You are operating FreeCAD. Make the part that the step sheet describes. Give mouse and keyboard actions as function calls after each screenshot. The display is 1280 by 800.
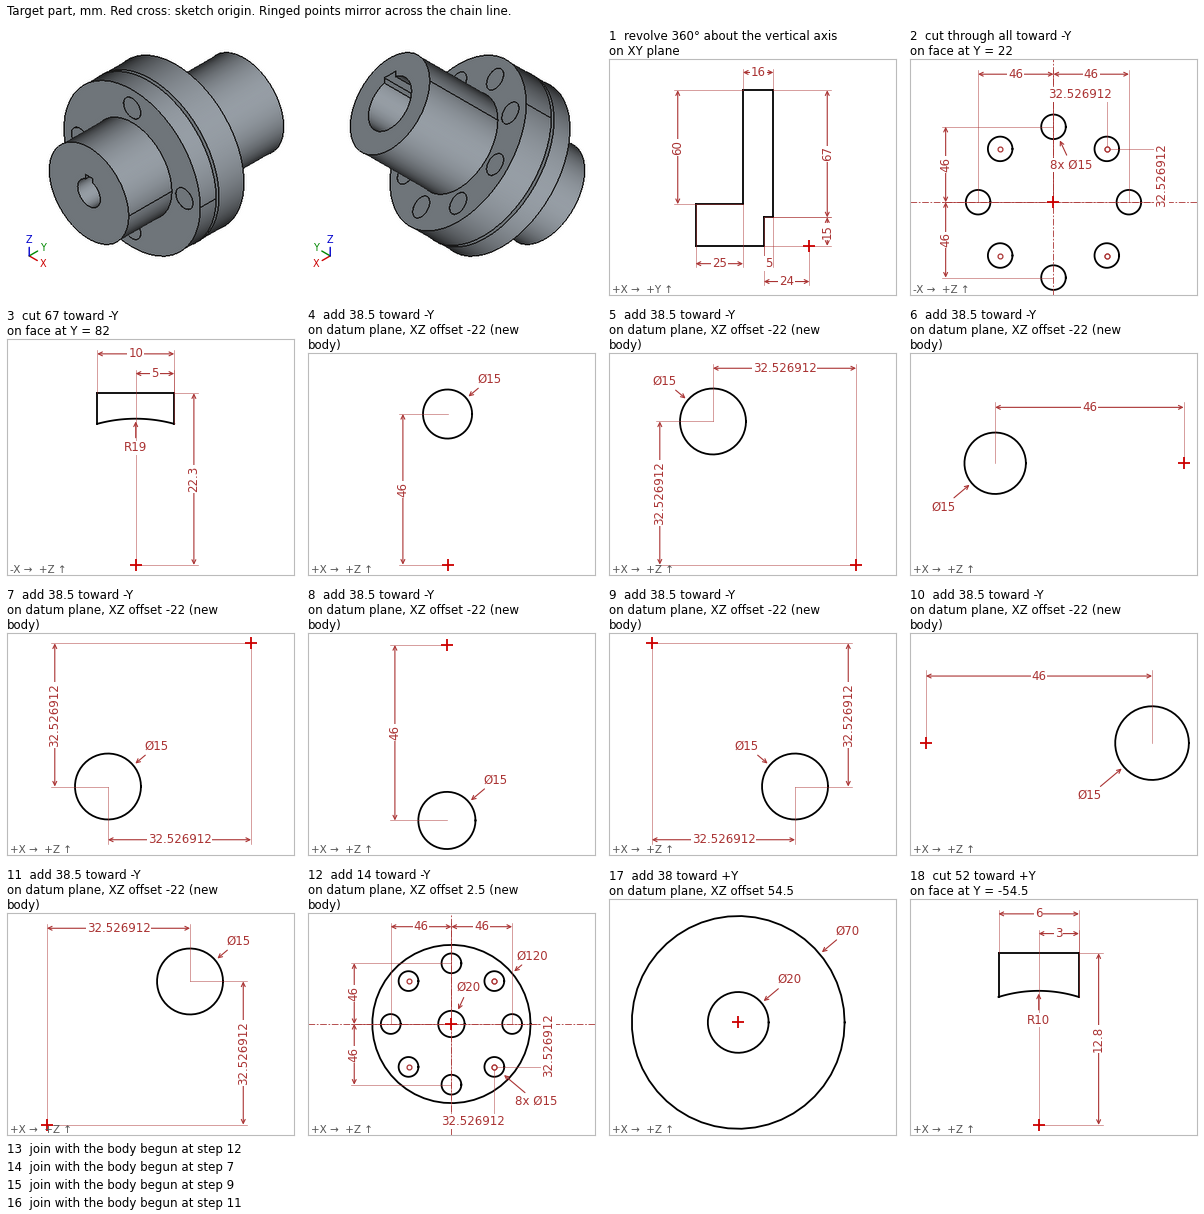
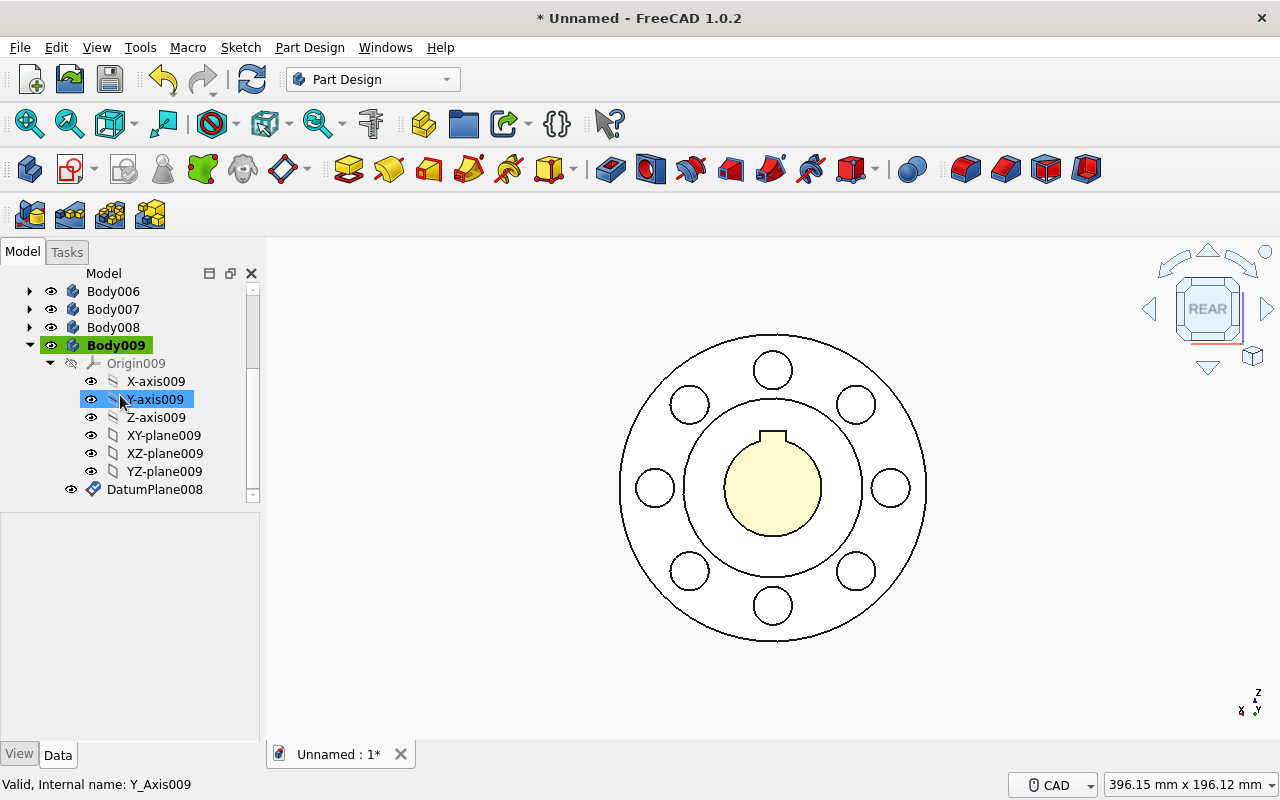
click(116, 489)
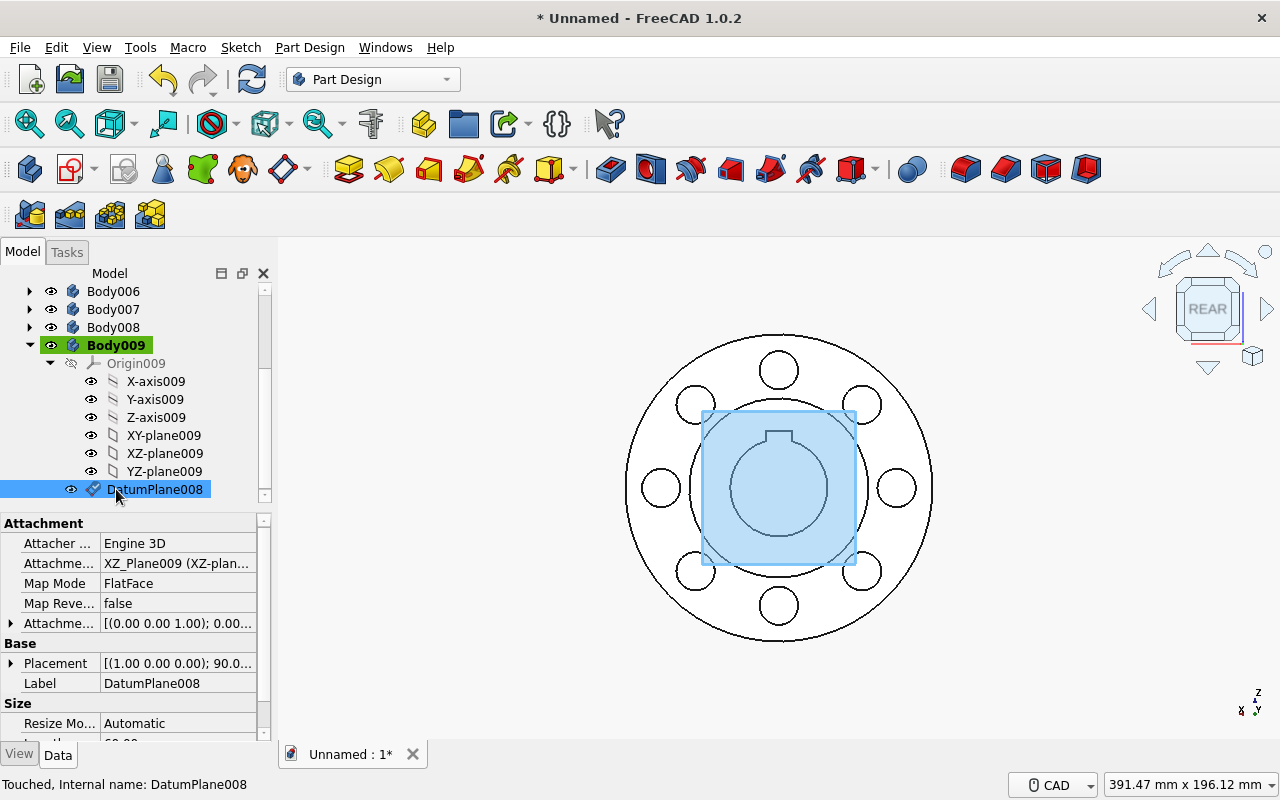
click(70, 170)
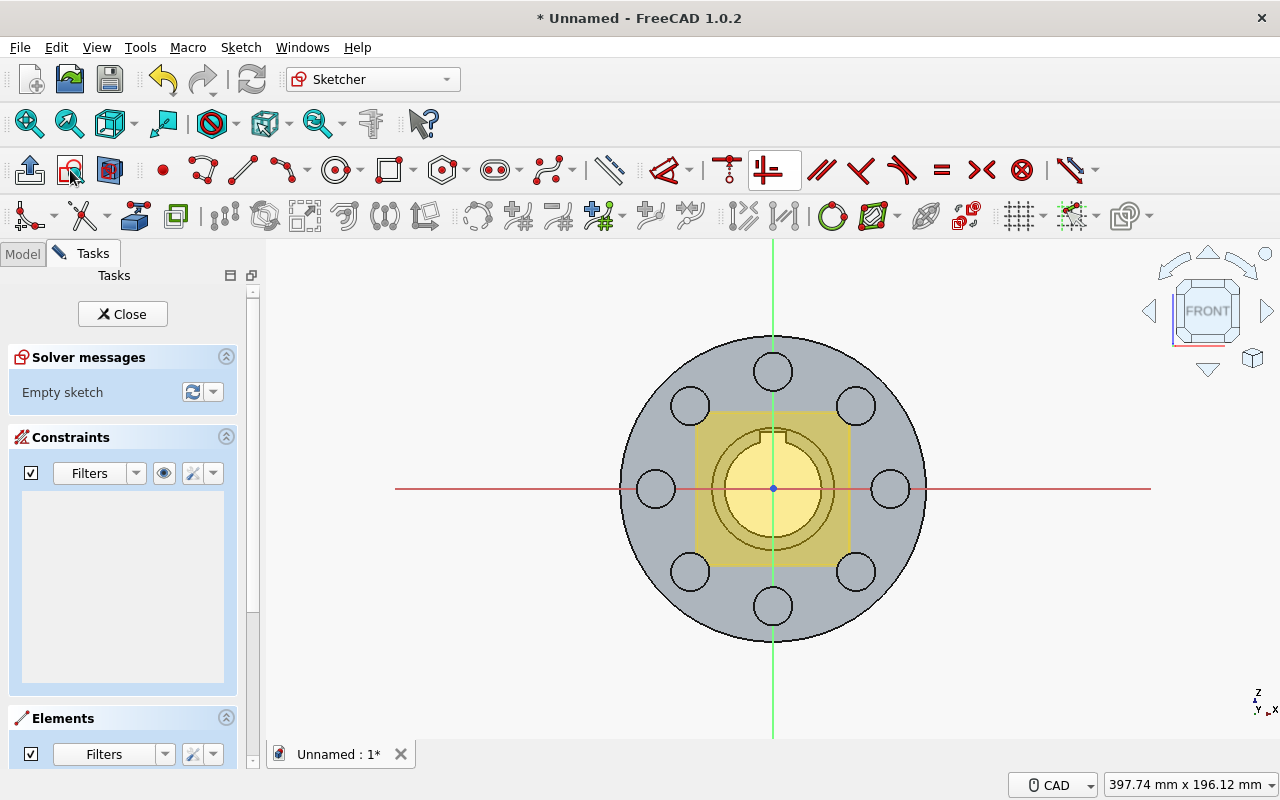
click(336, 170)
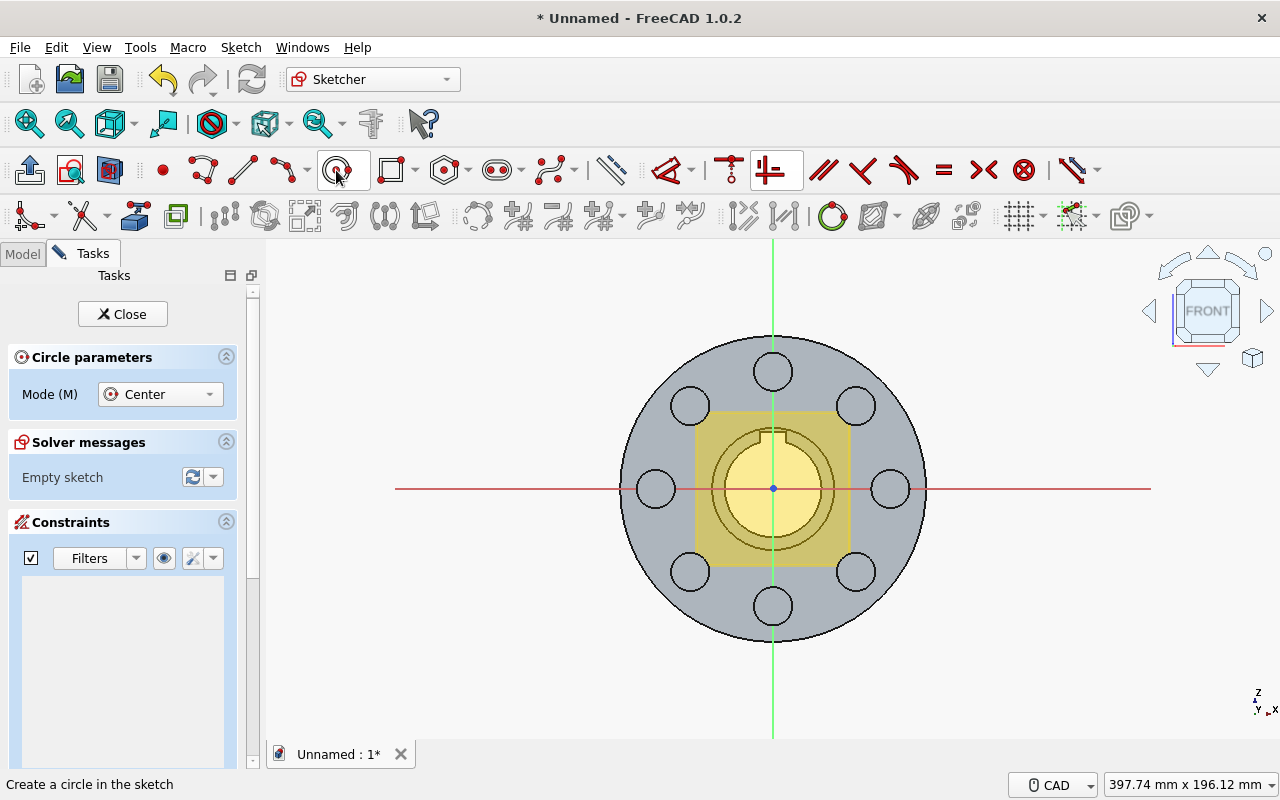
click(773, 489)
click(881, 381)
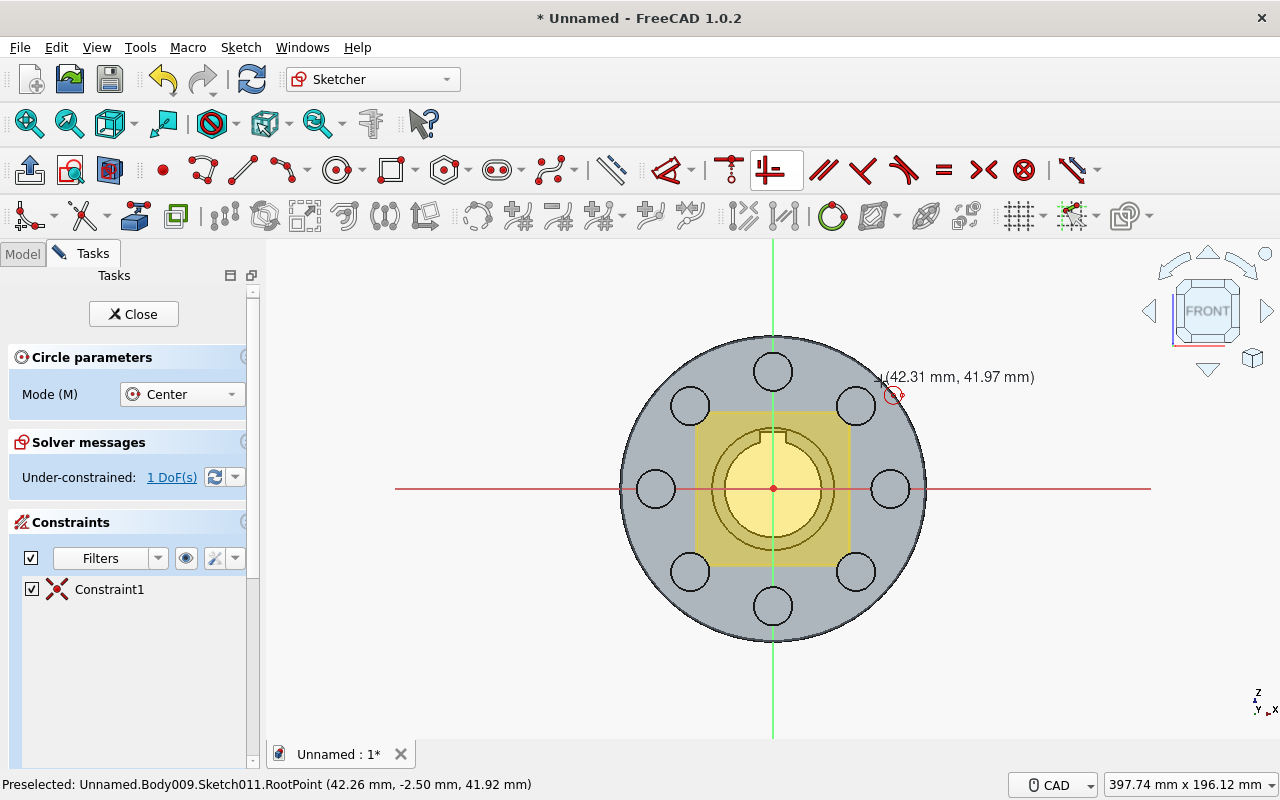
click(856, 572)
click(870, 558)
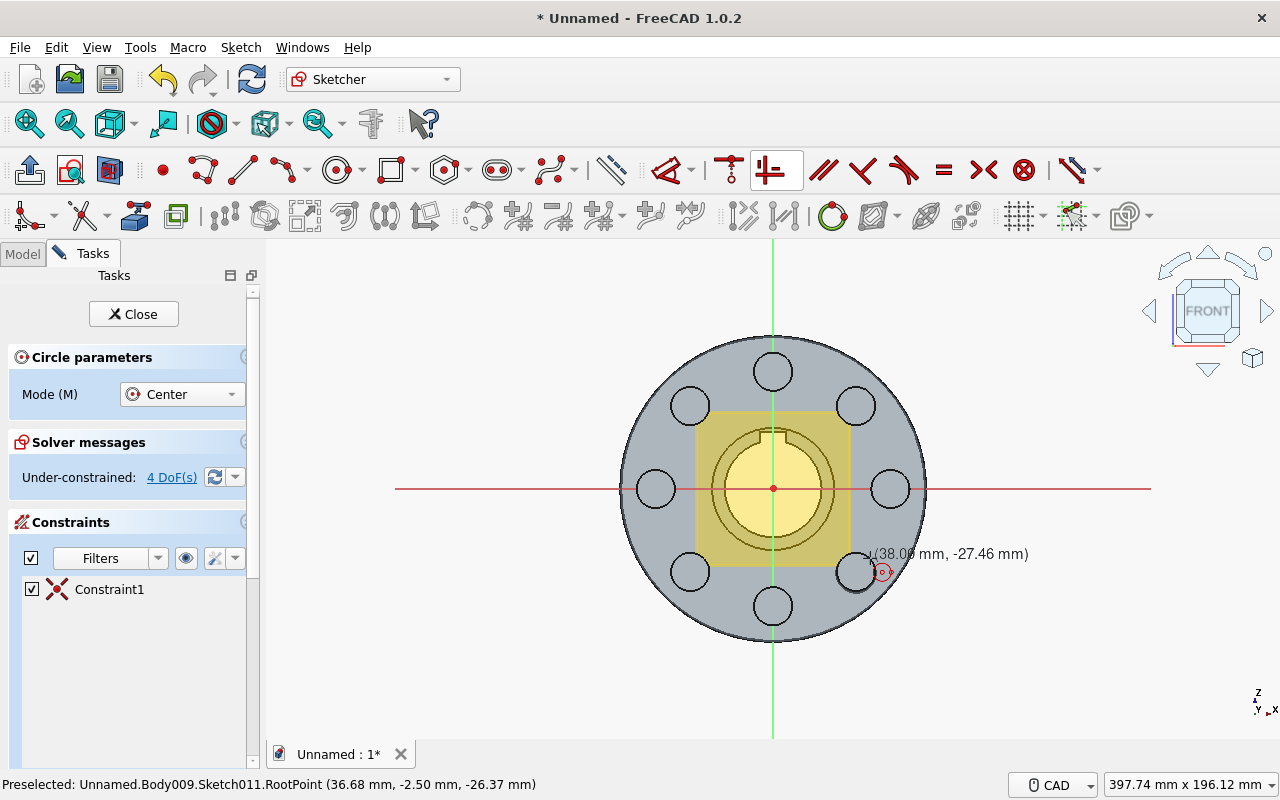
click(773, 606)
click(791, 600)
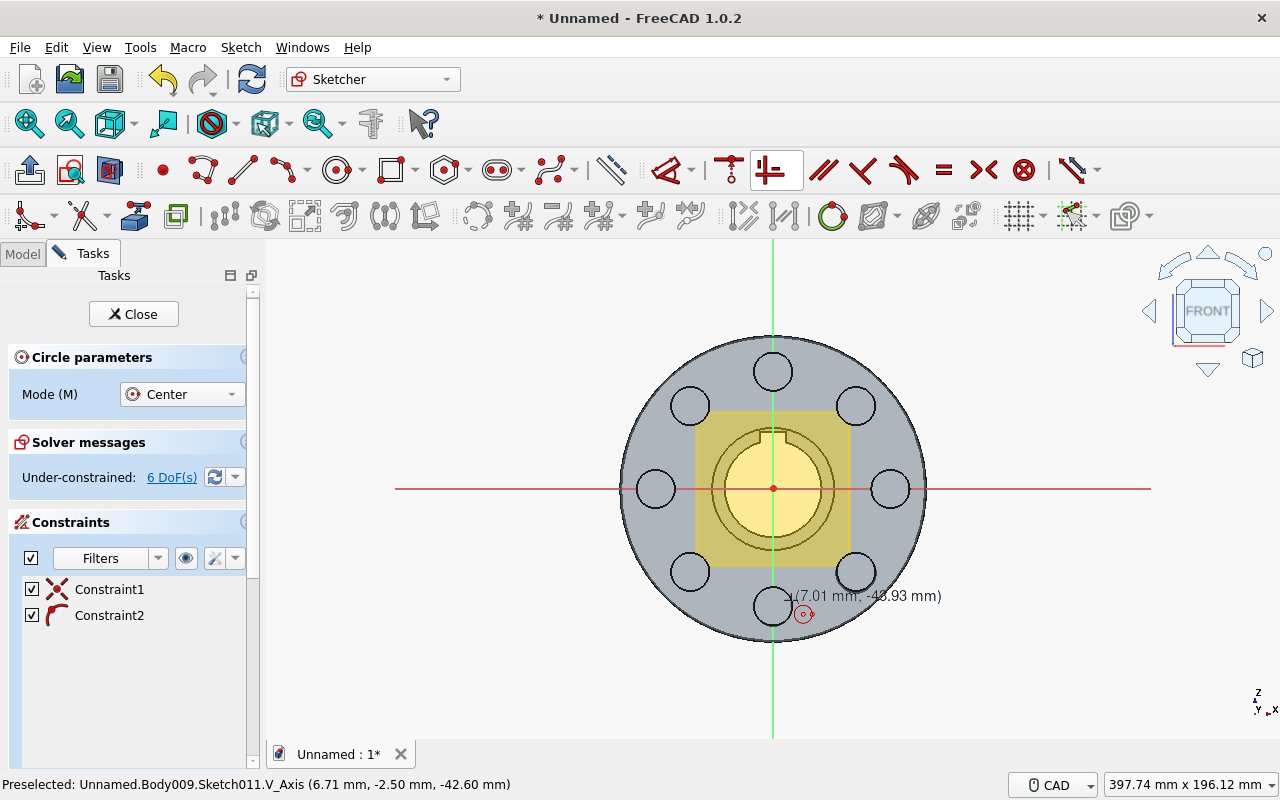
click(773, 489)
click(791, 471)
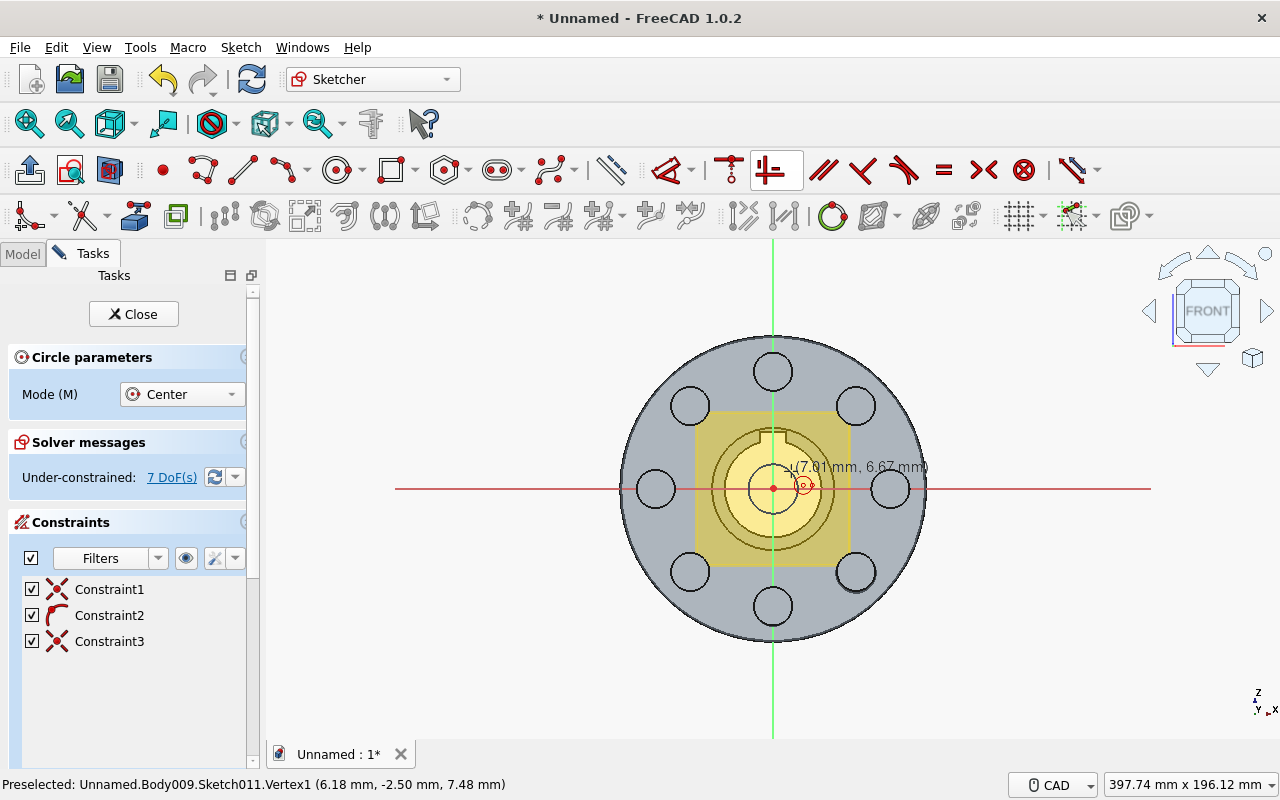
click(890, 489)
click(897, 471)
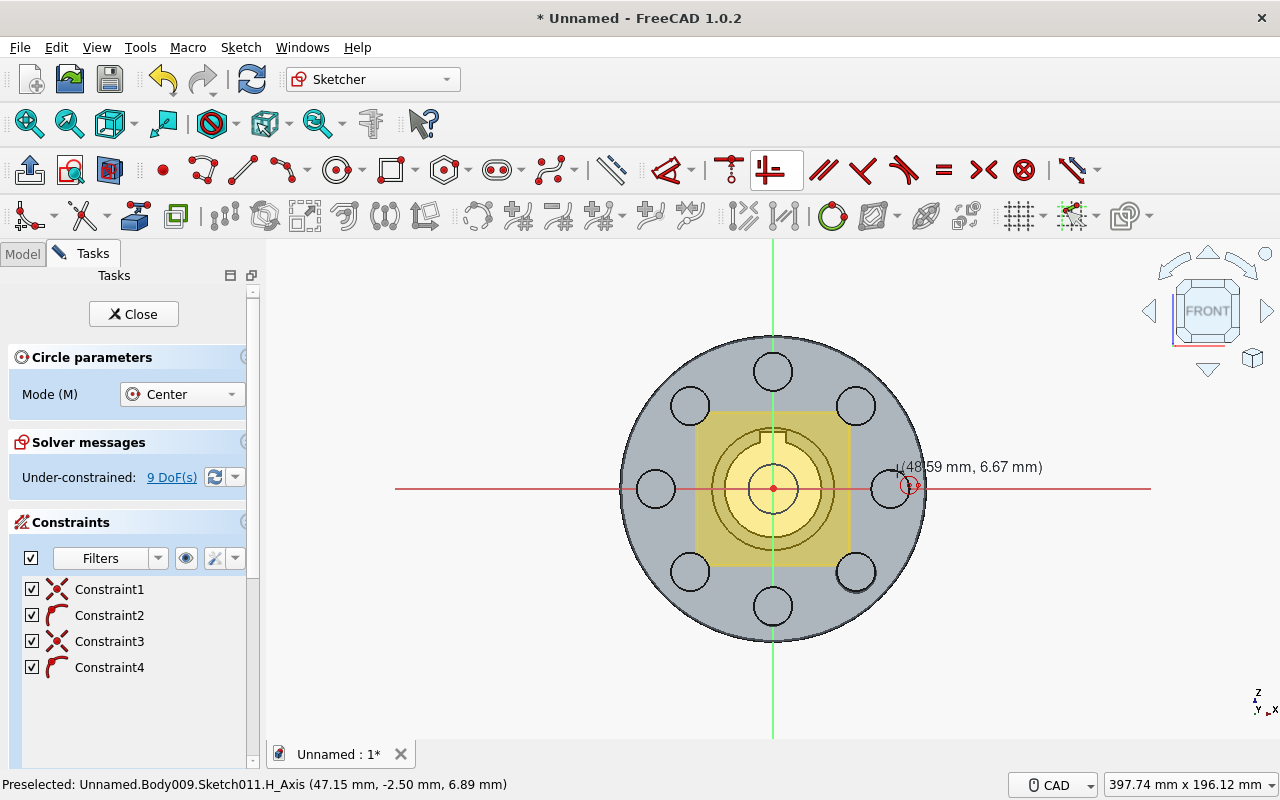
click(856, 406)
click(870, 393)